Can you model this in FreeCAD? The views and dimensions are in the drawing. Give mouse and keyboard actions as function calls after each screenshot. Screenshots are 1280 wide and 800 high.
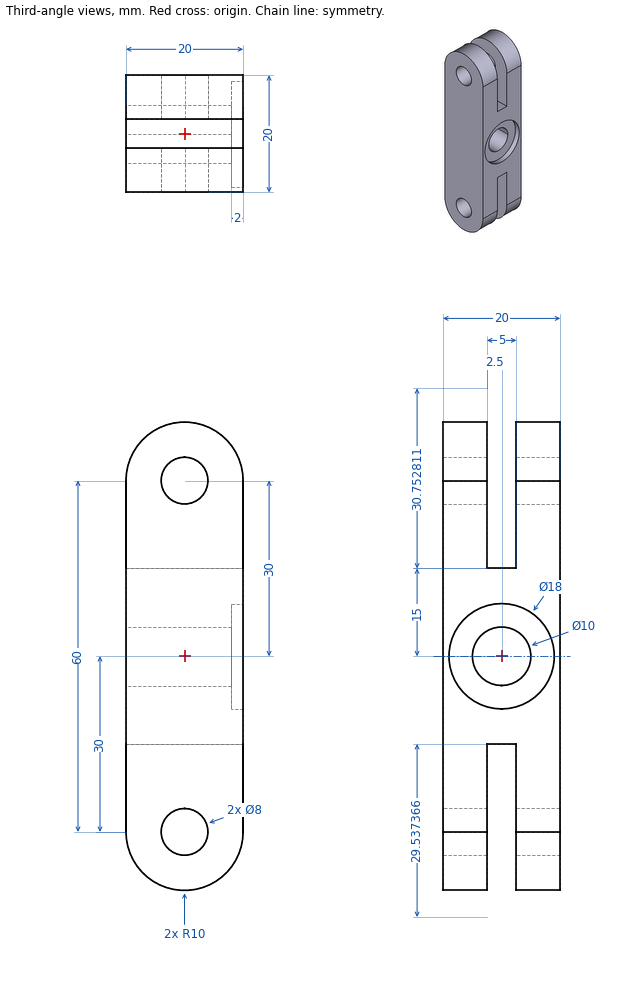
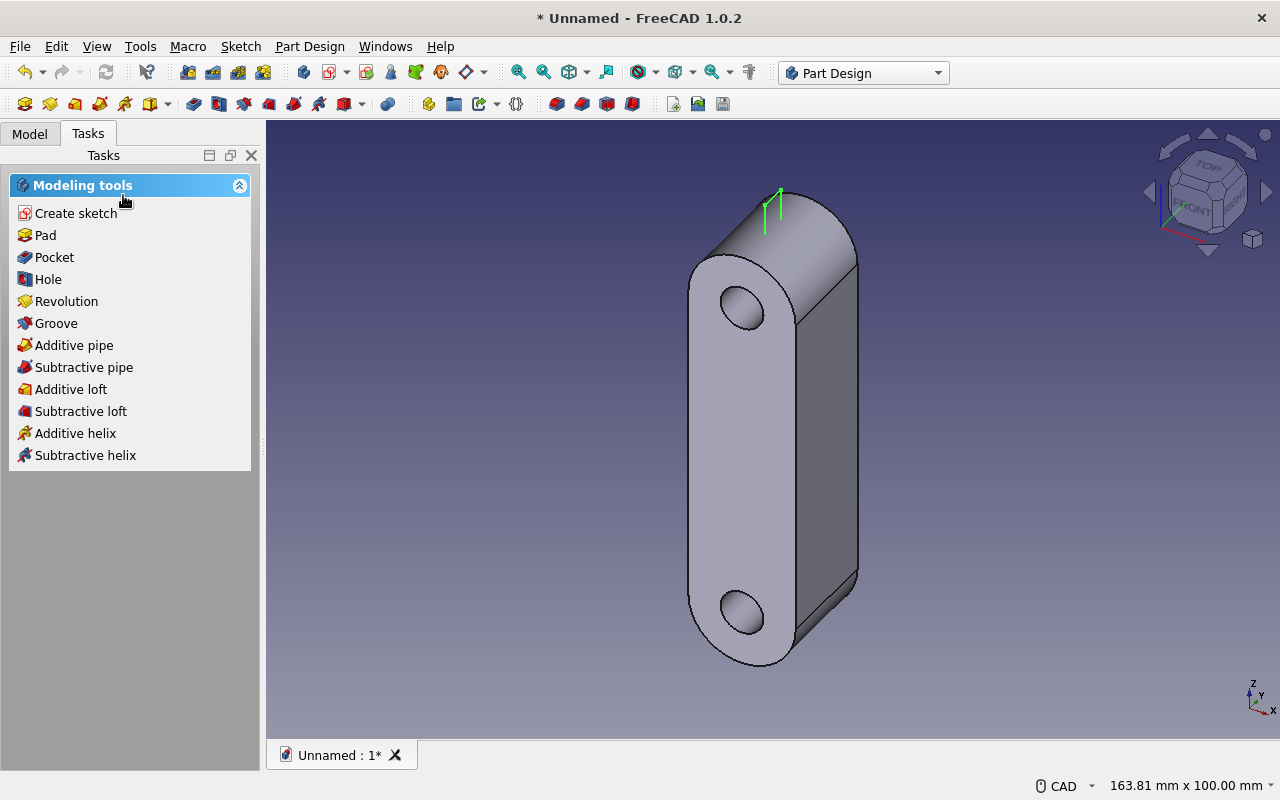
click(194, 104)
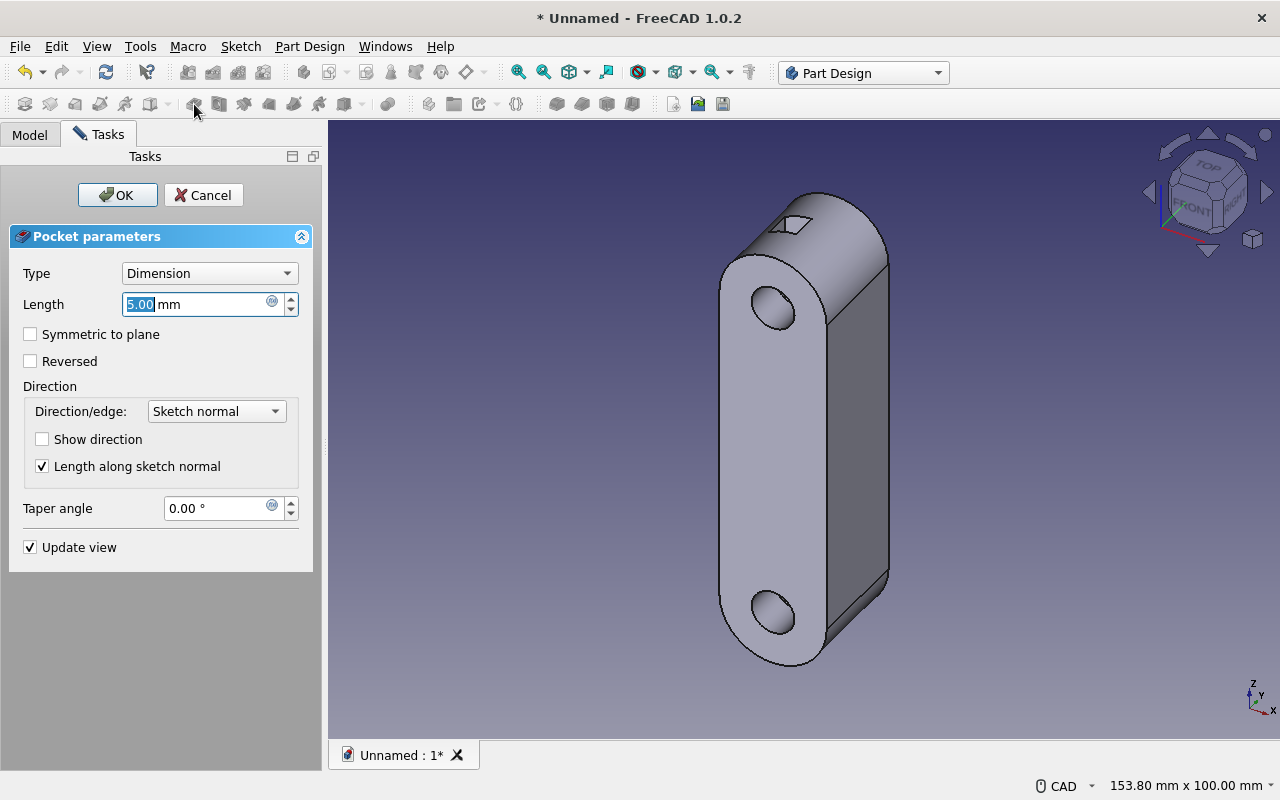
text(20)
key(Tab)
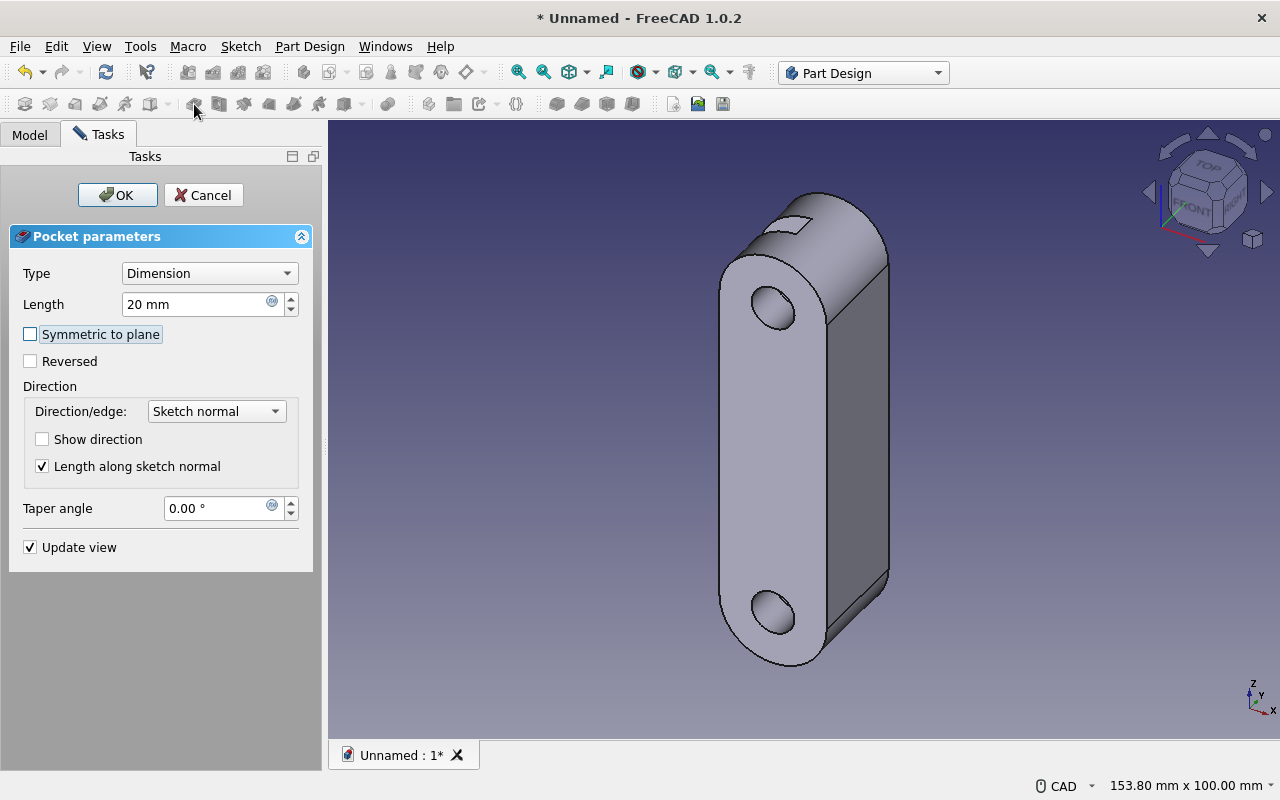
click(31, 334)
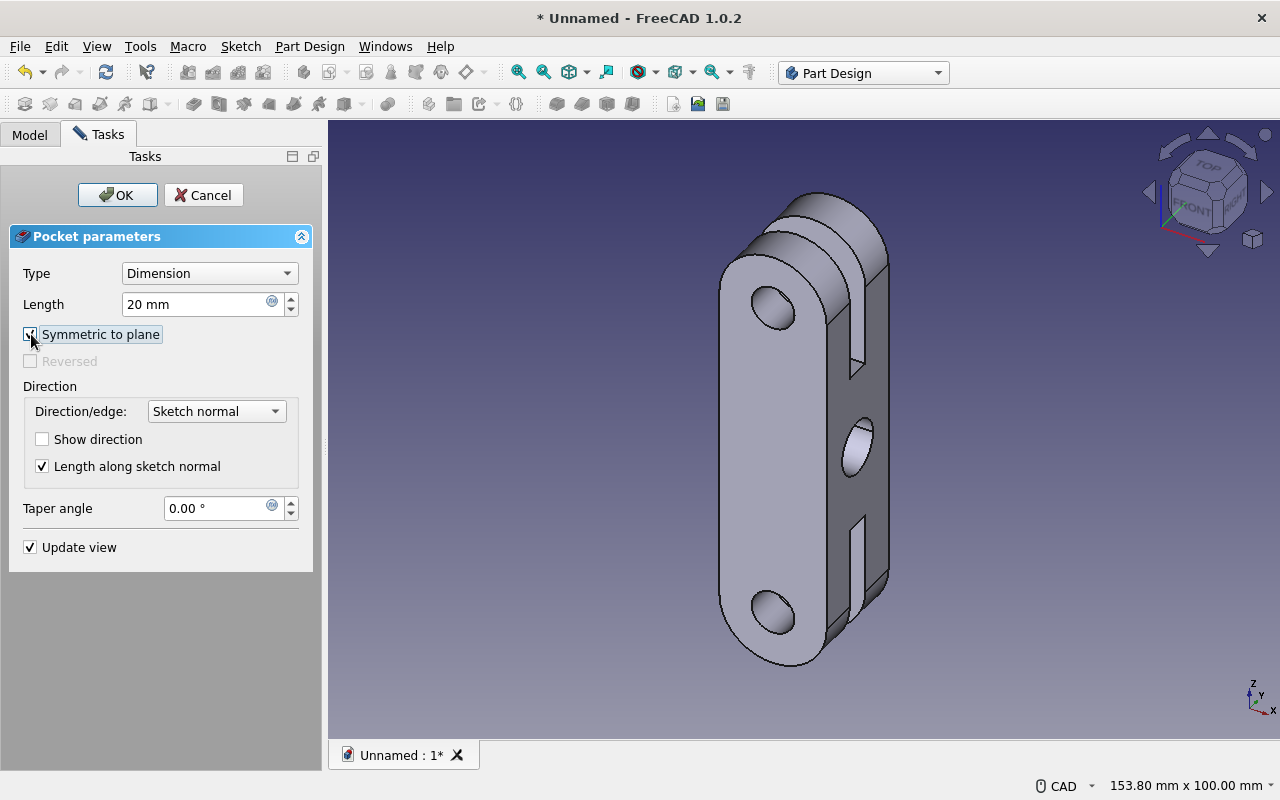
click(118, 195)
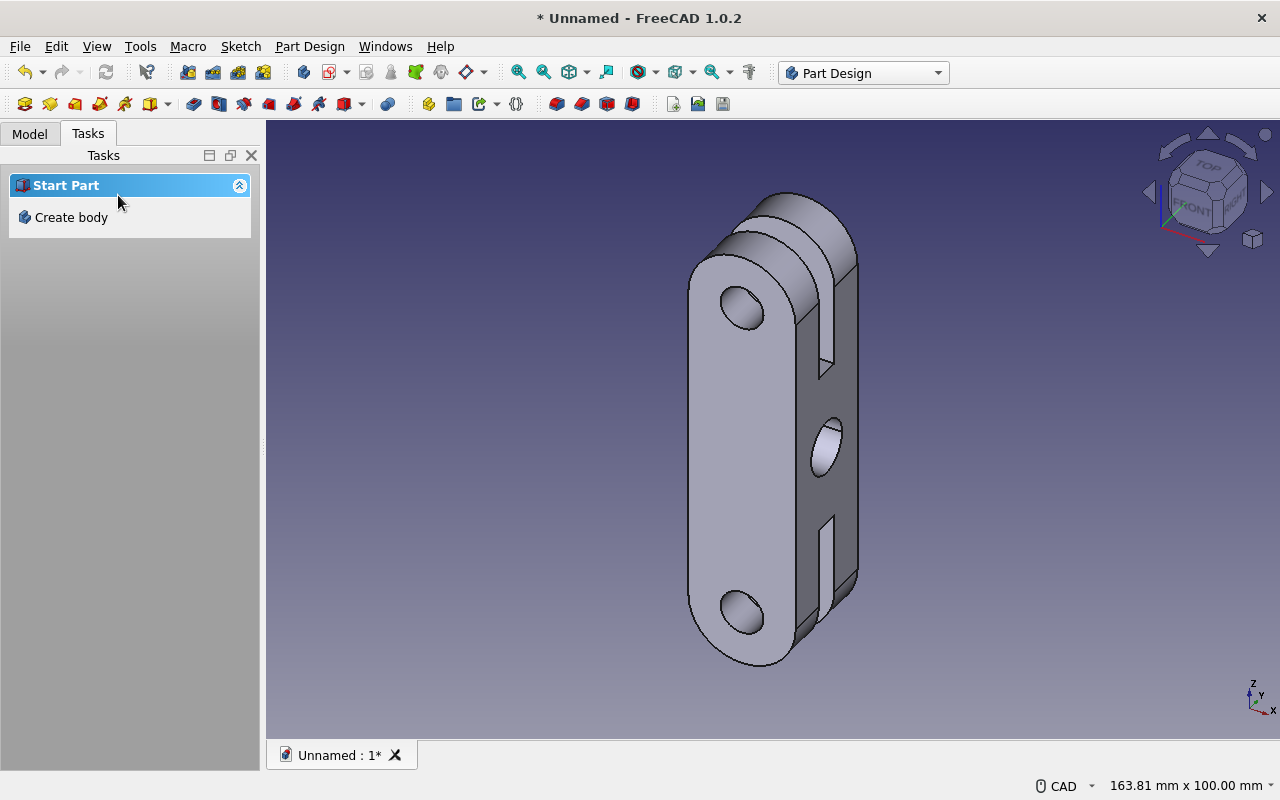
click(844, 385)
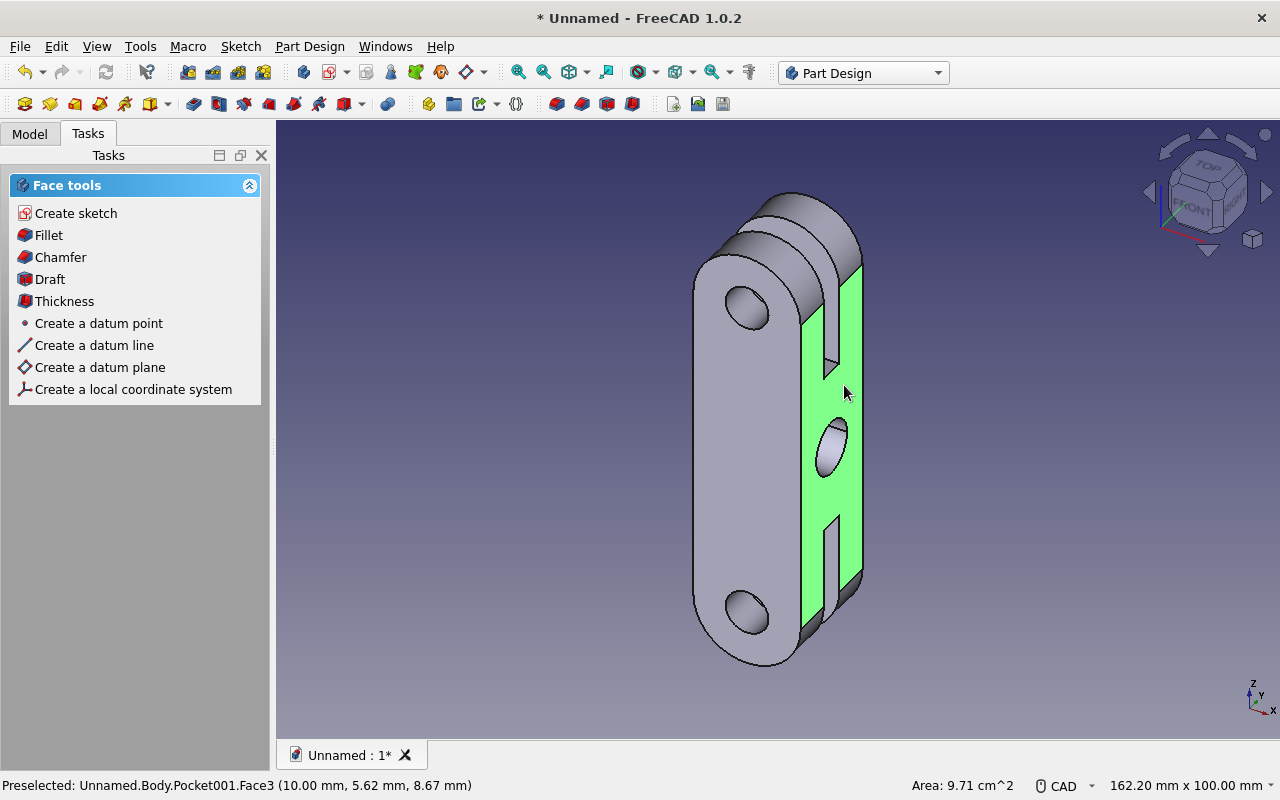
click(328, 72)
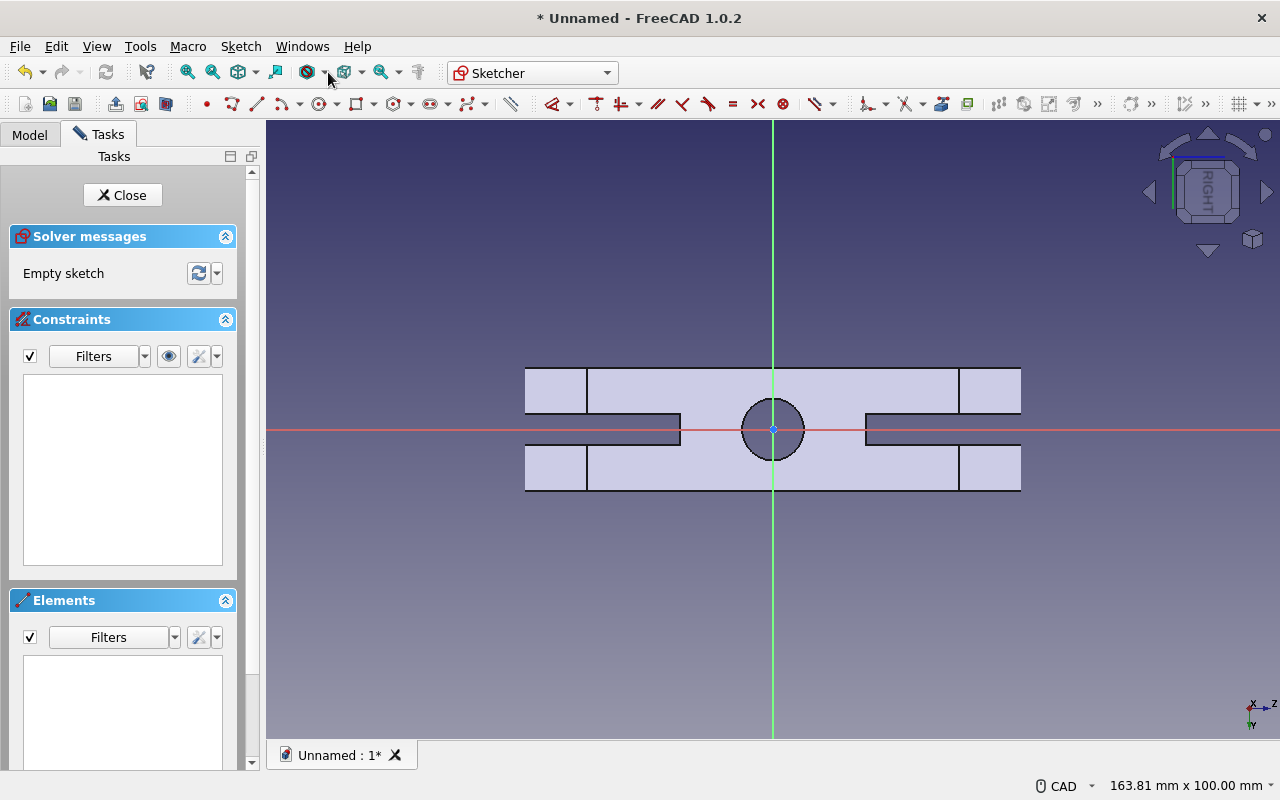
scroll(803, 430, up, 6)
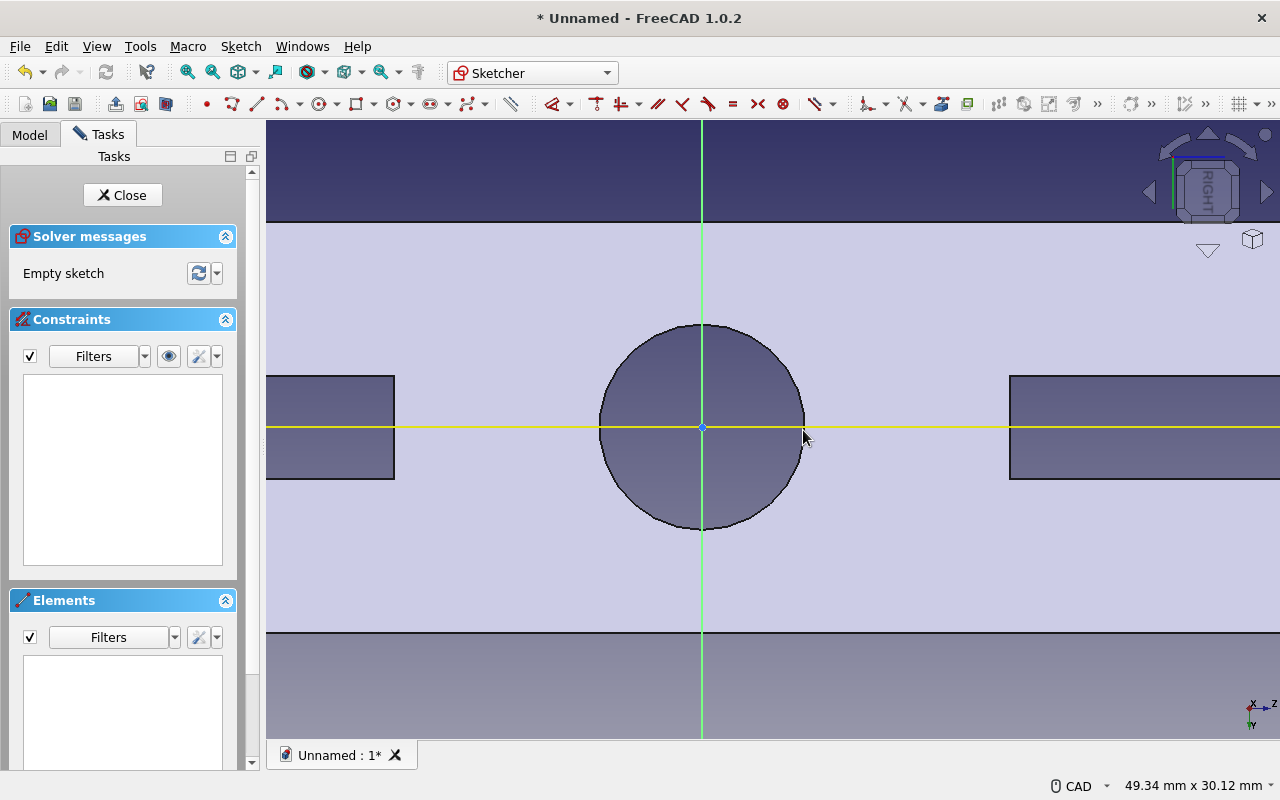
click(318, 104)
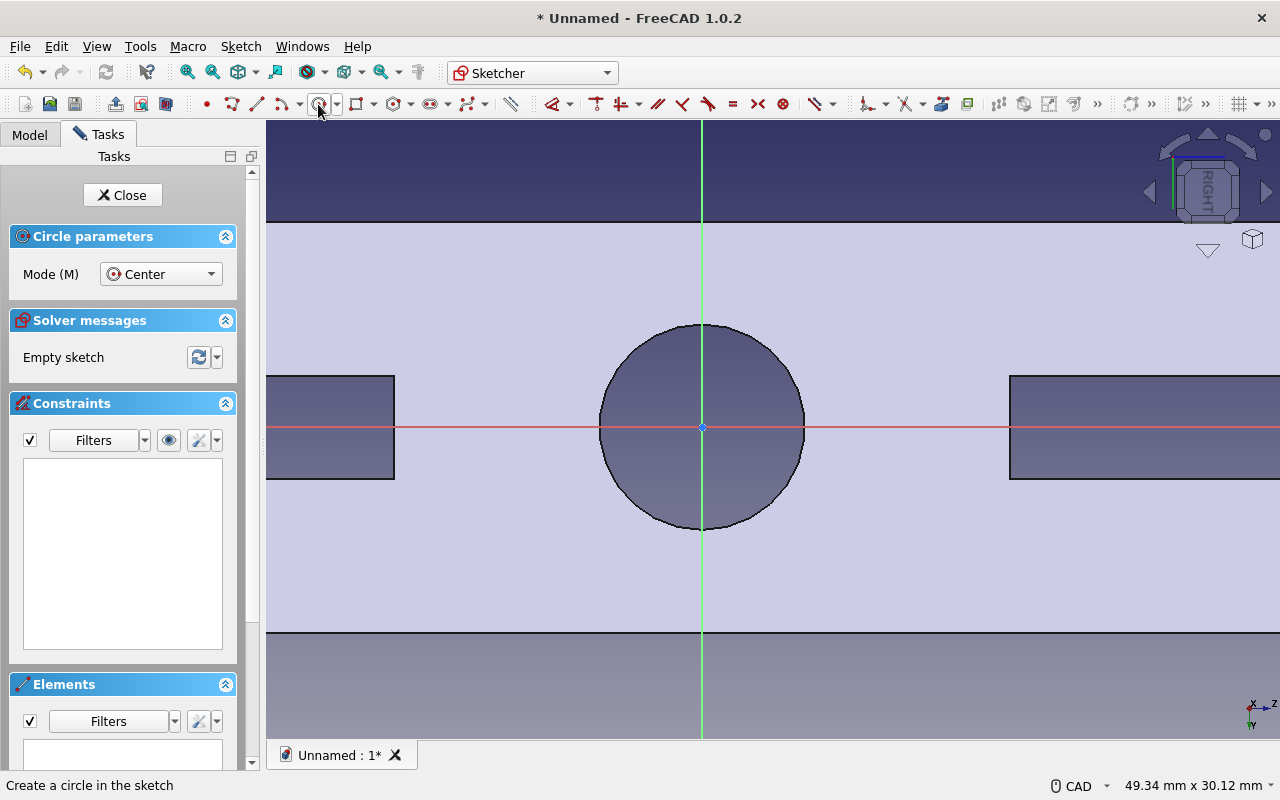
click(702, 427)
click(833, 296)
key(Escape)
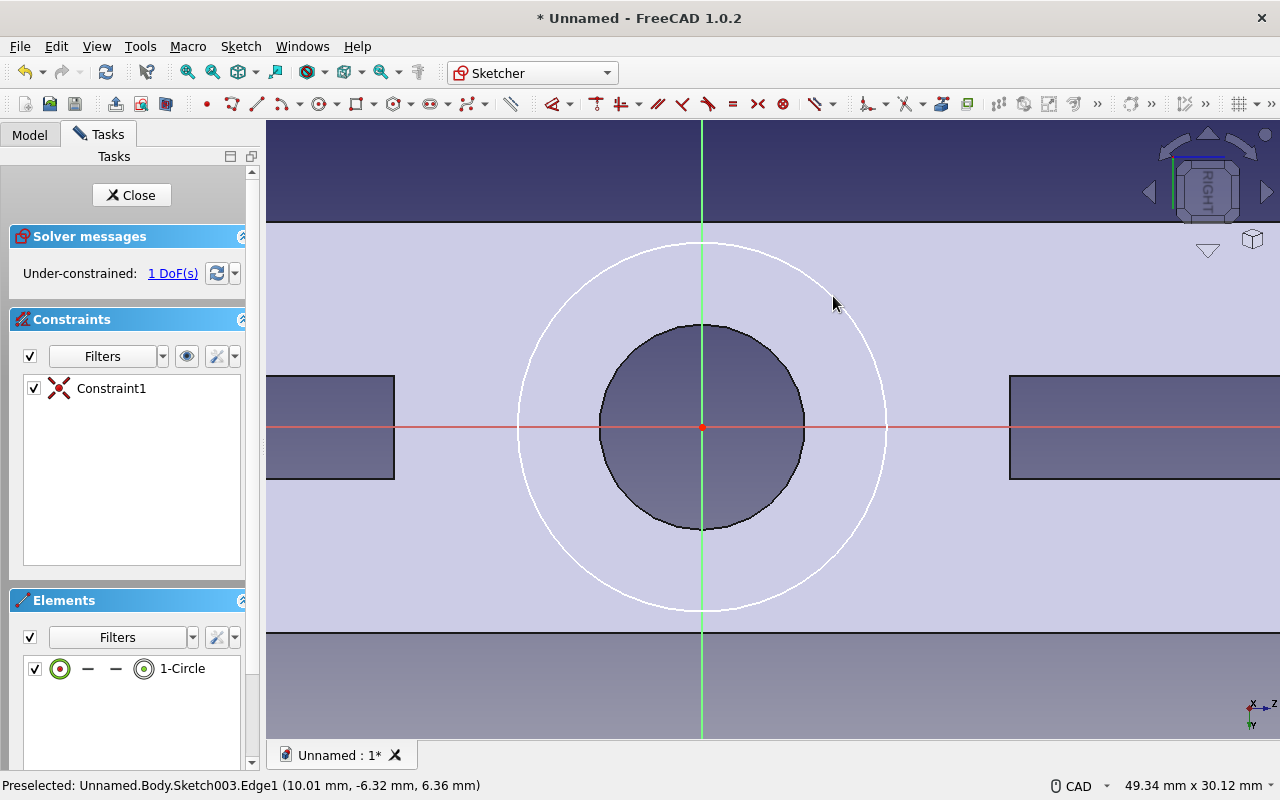
click(552, 104)